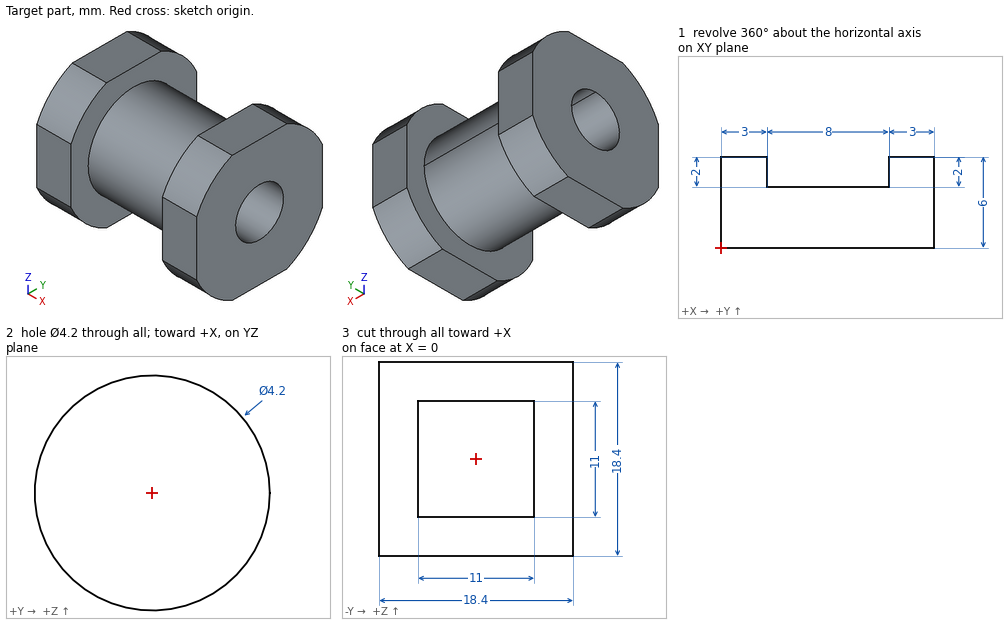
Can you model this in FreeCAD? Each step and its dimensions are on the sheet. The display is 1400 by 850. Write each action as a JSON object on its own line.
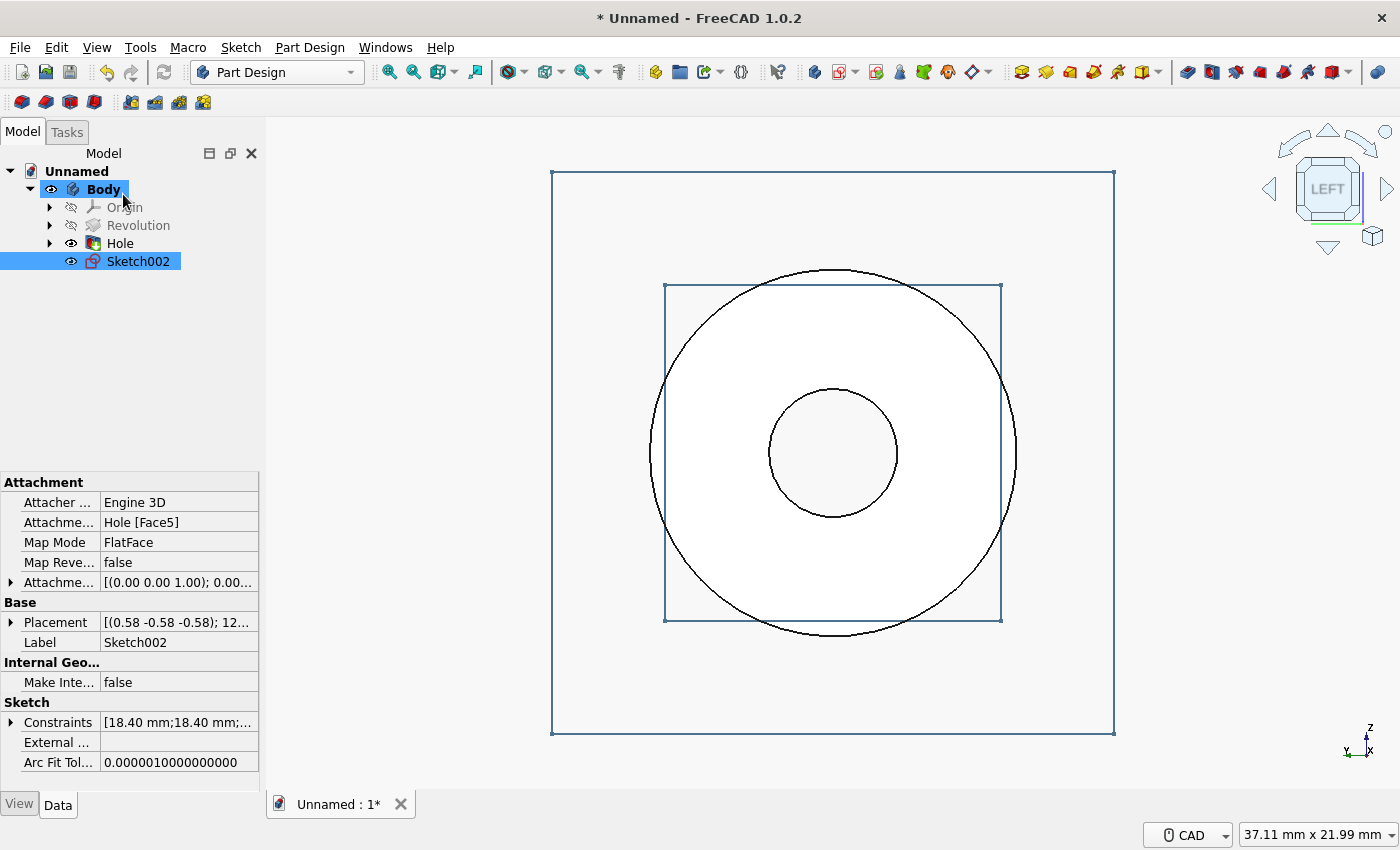
{"action": "left_click", "coordinate": [1188, 72]}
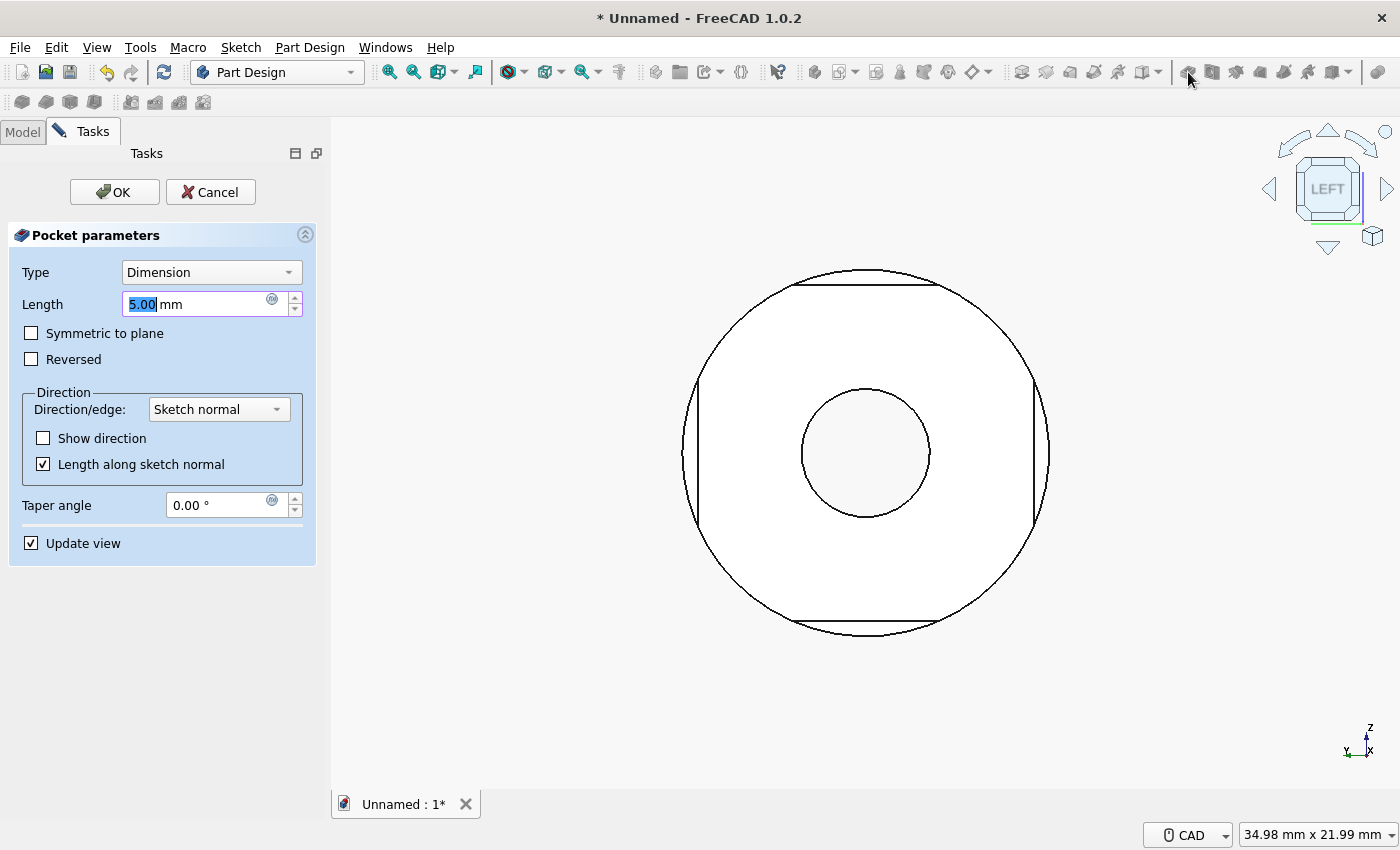
{"action": "left_click", "coordinate": [212, 272]}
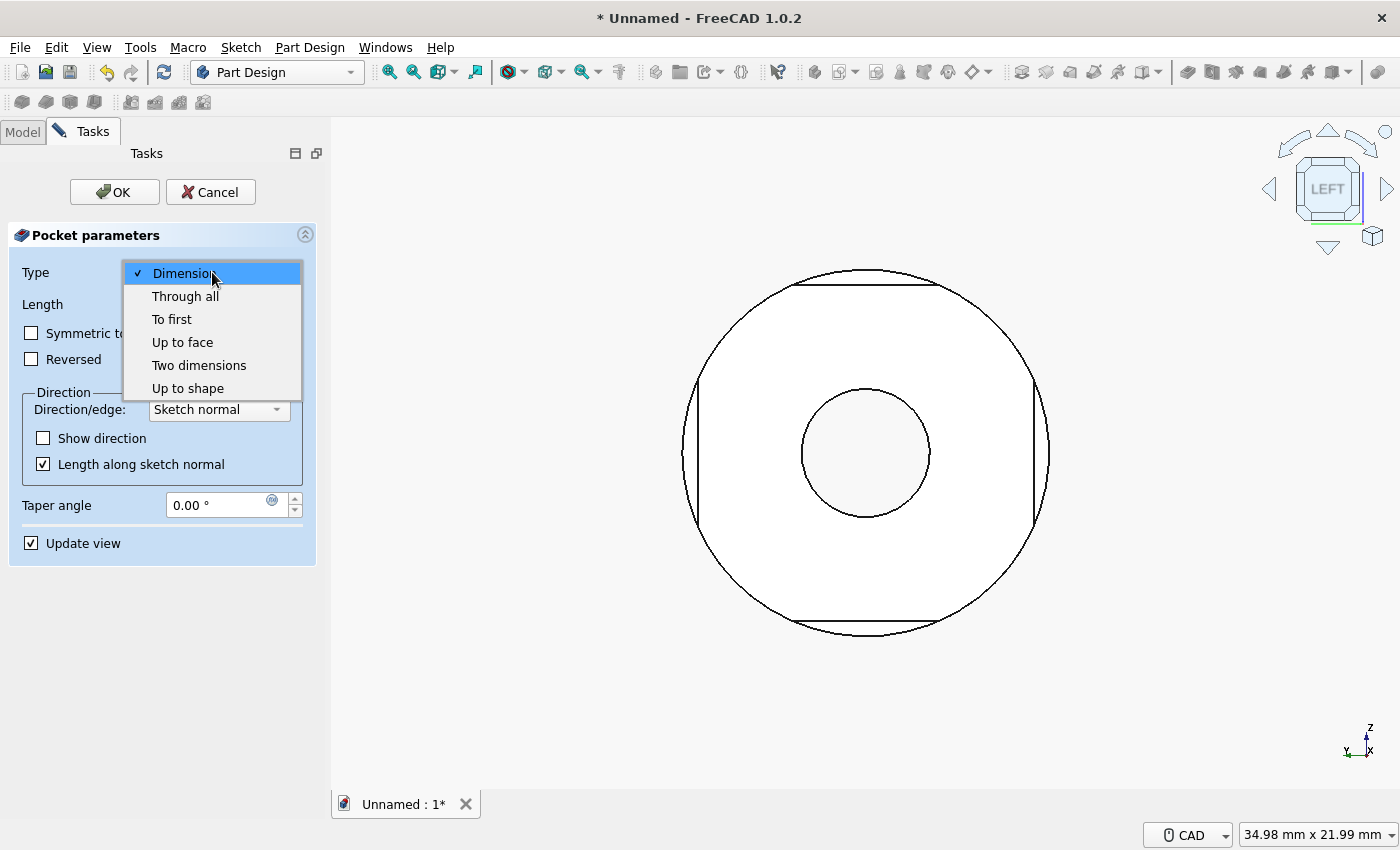
{"action": "left_click", "coordinate": [212, 296]}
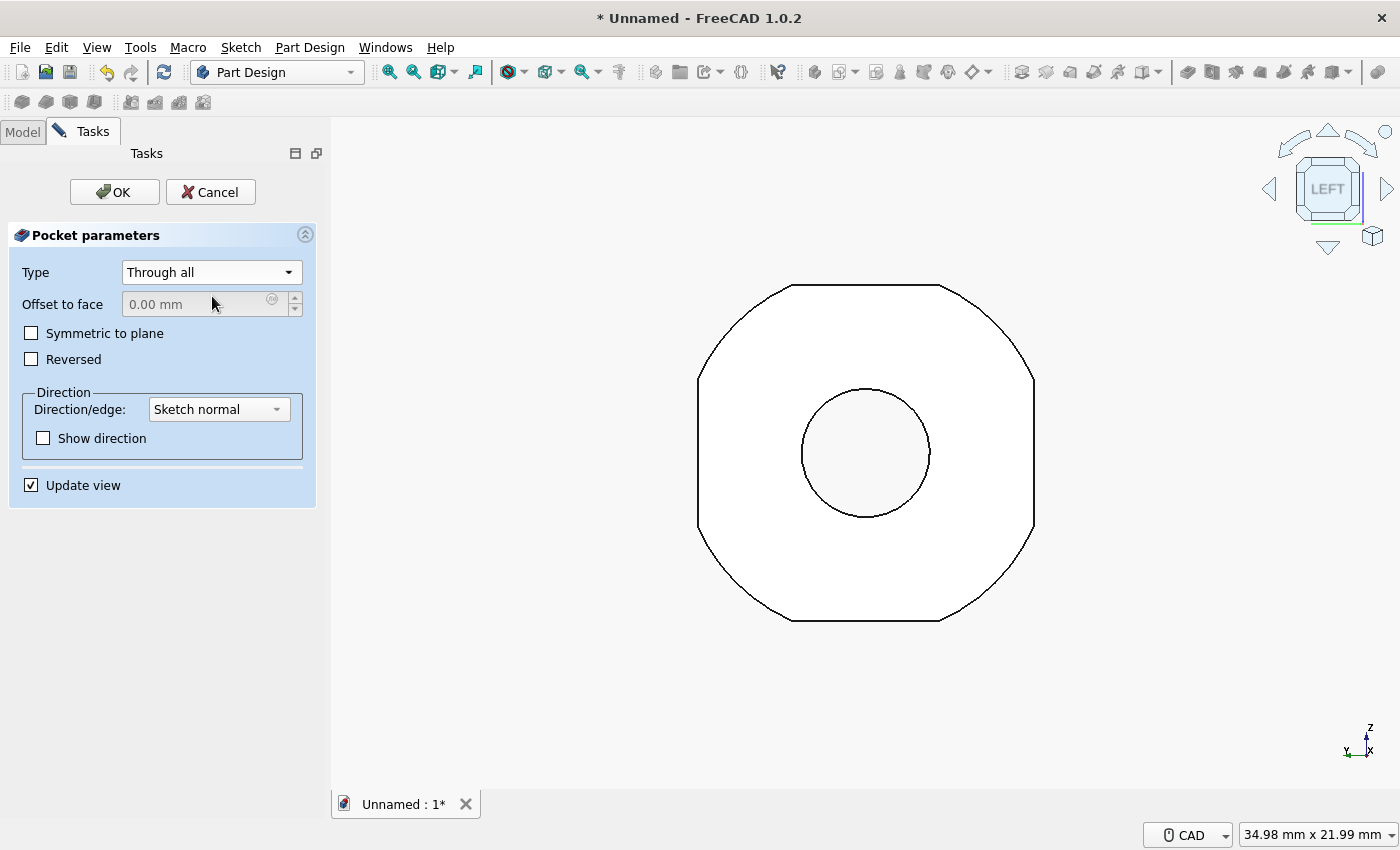
{"action": "left_click", "coordinate": [115, 192]}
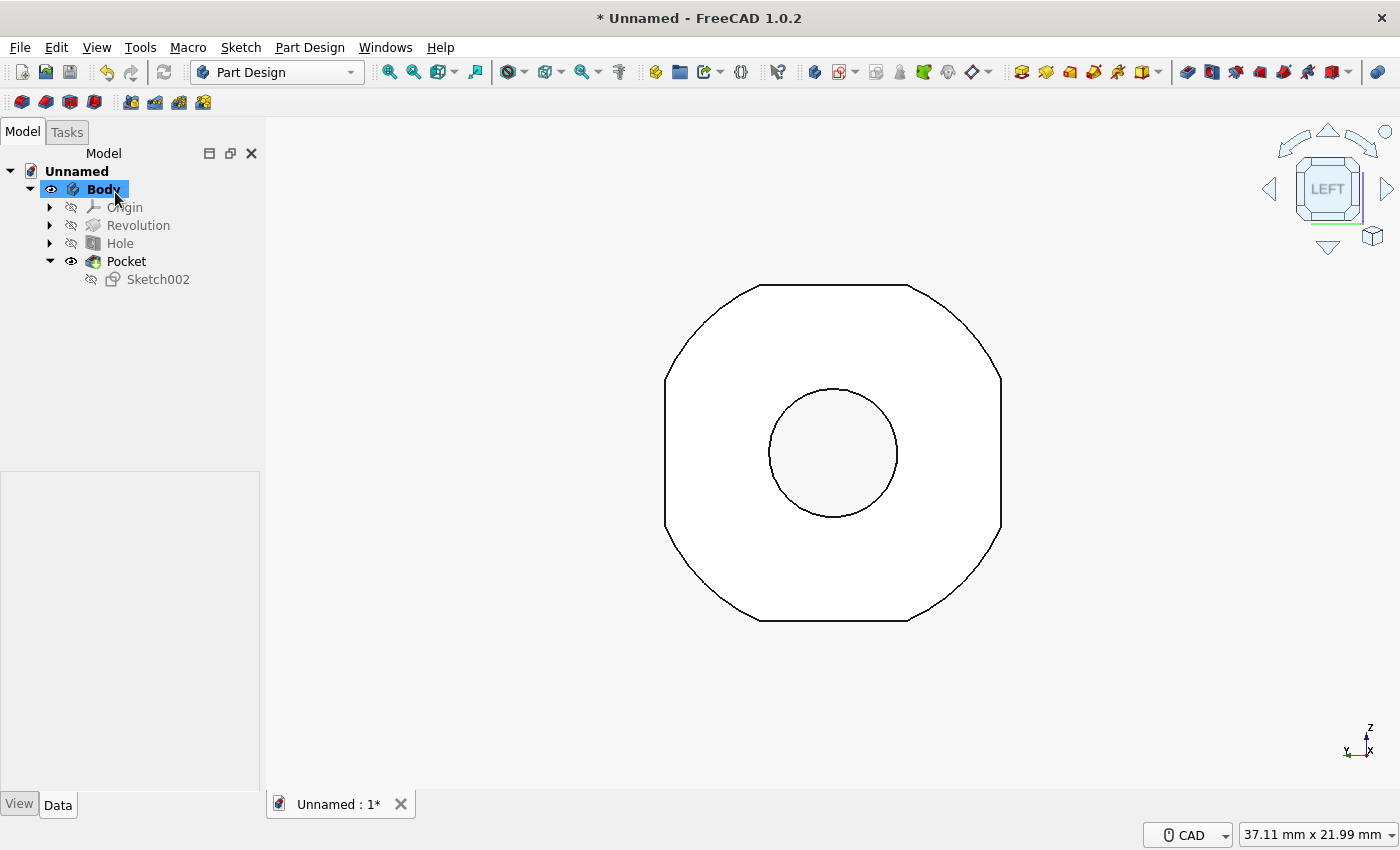
{"action": "key", "text": "0"}